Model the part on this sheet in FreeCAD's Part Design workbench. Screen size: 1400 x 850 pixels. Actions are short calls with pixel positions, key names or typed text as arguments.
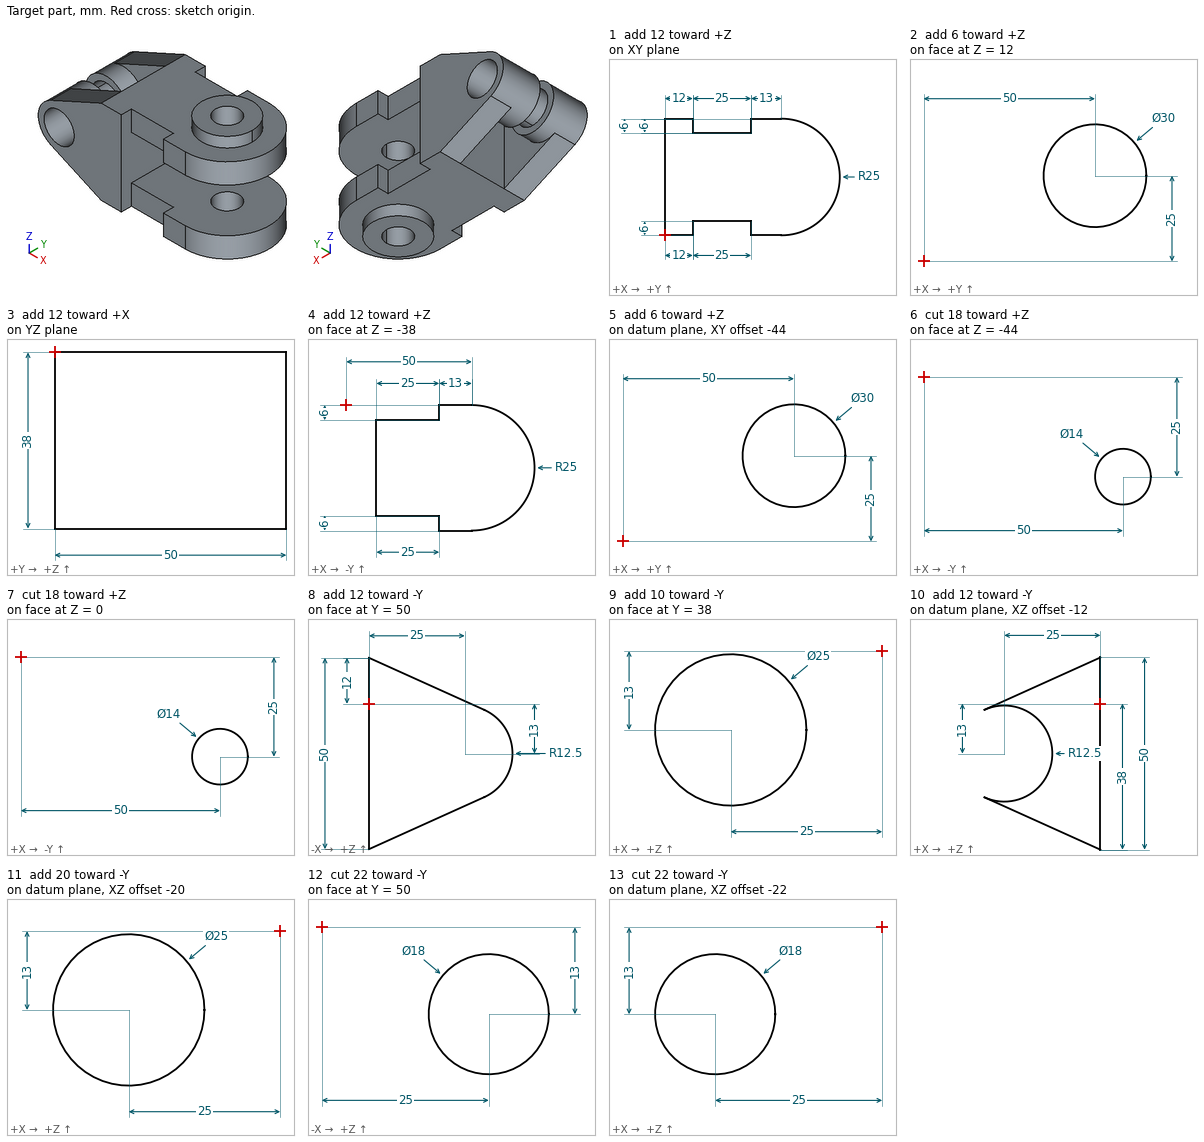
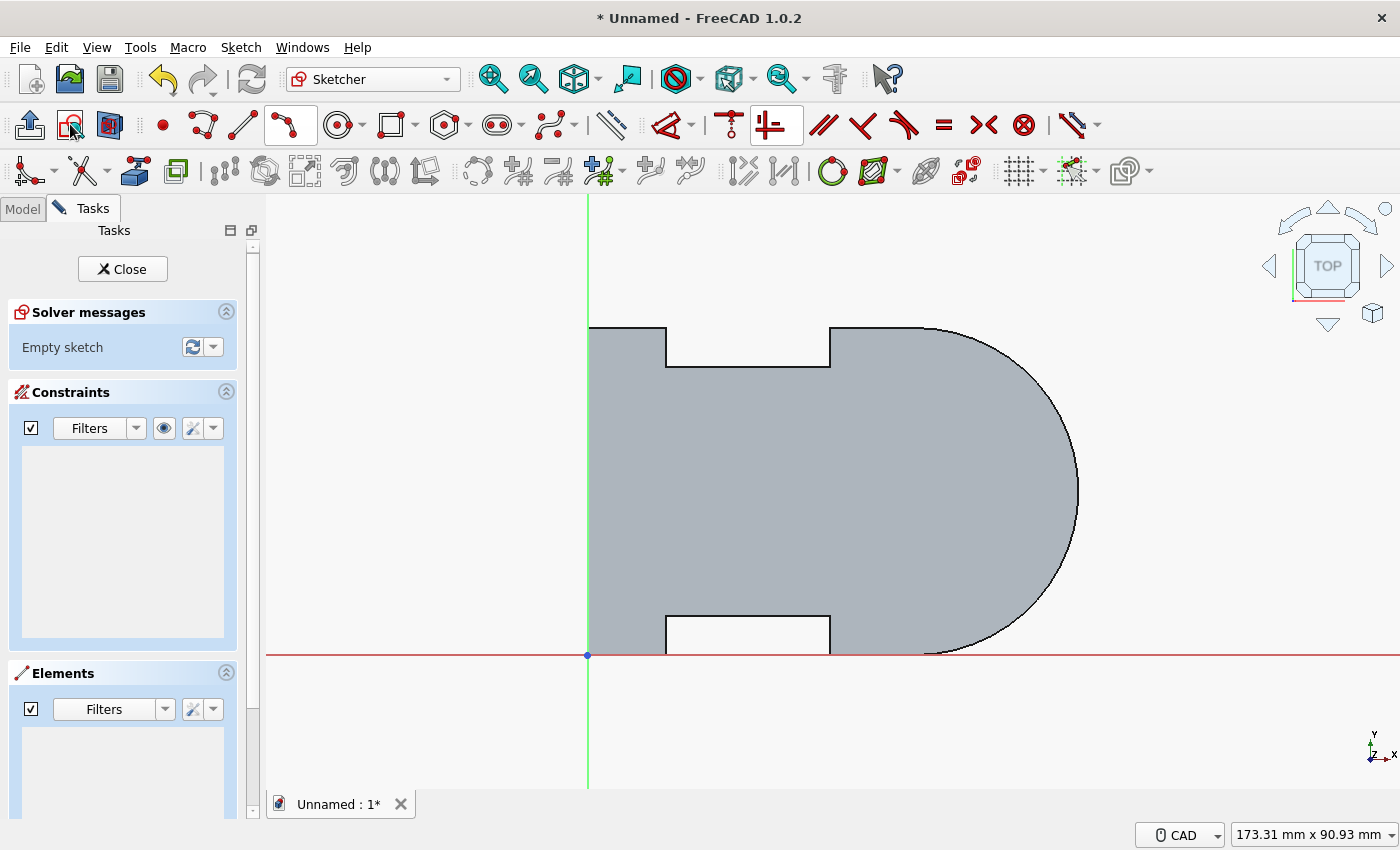
scroll(873, 591, up, 2)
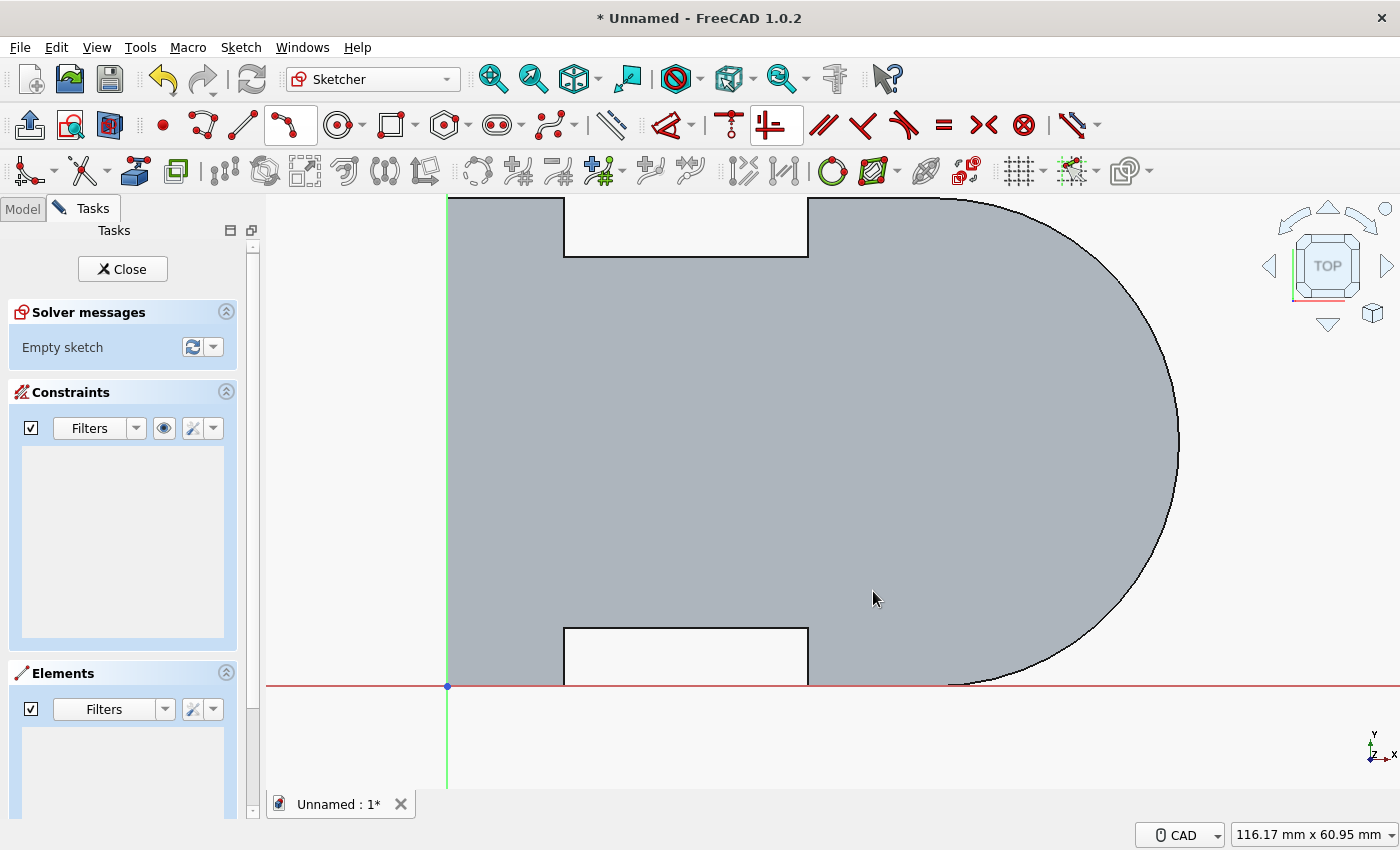
click(338, 126)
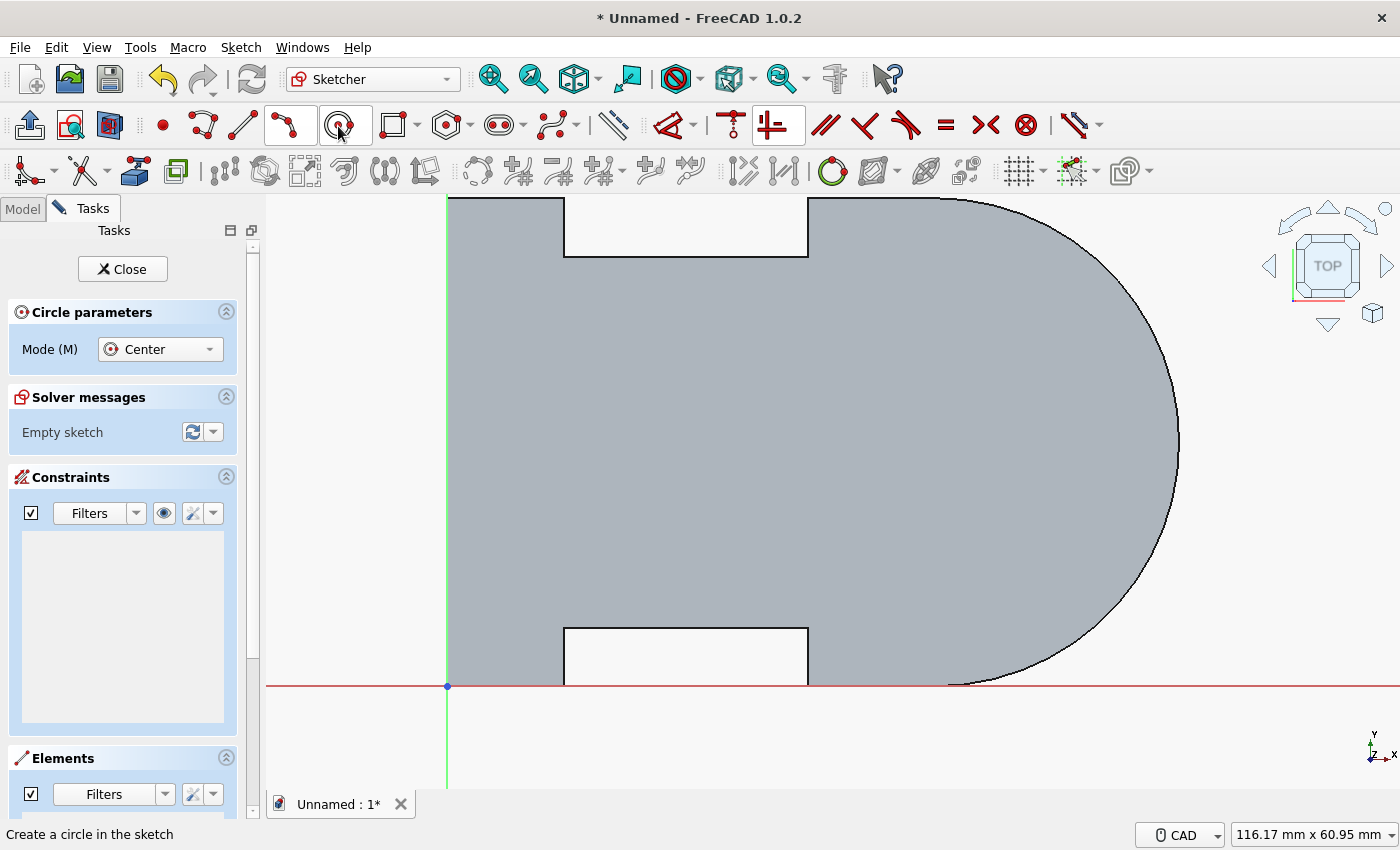
click(935, 442)
click(1039, 339)
key(Escape)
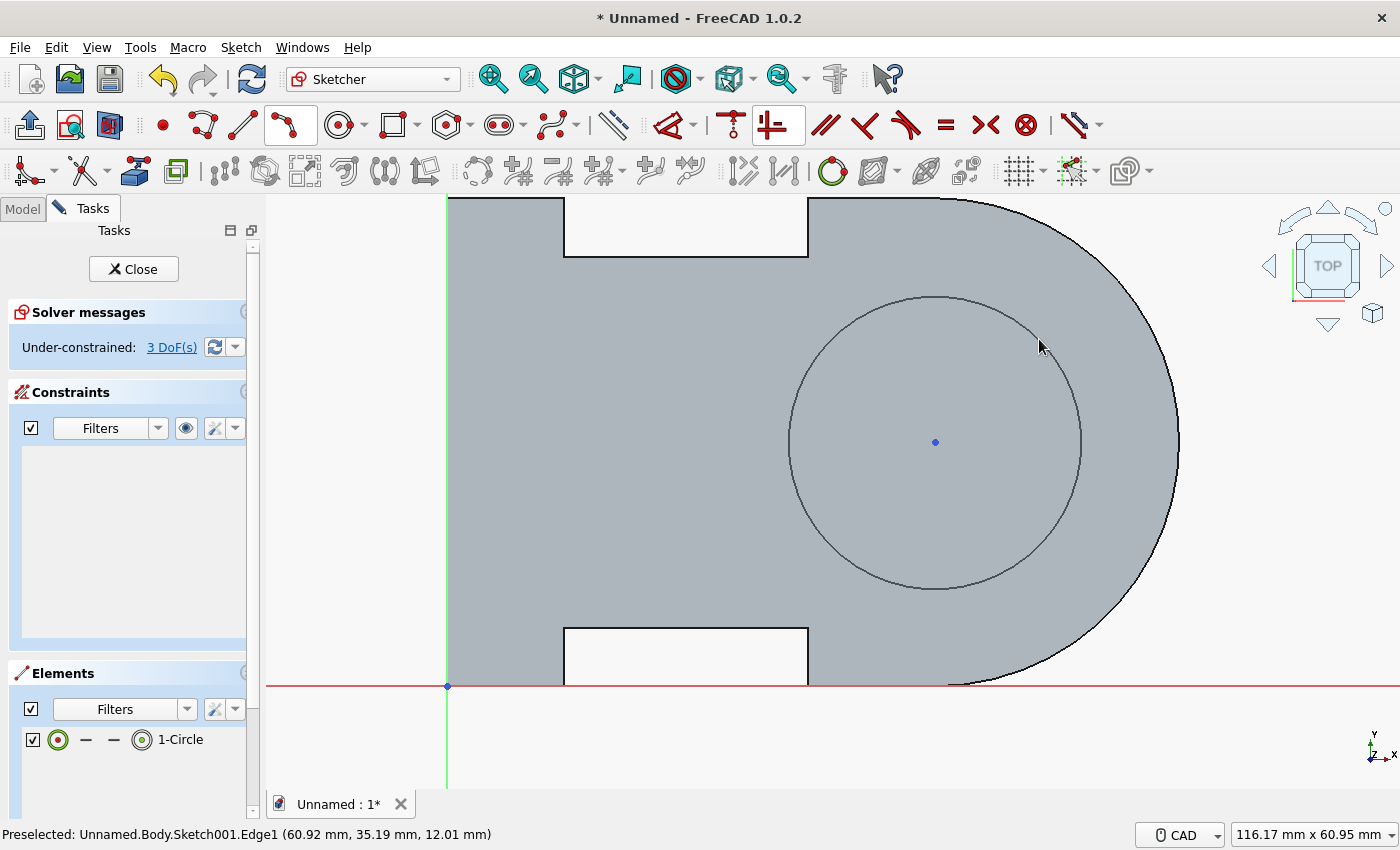
click(668, 126)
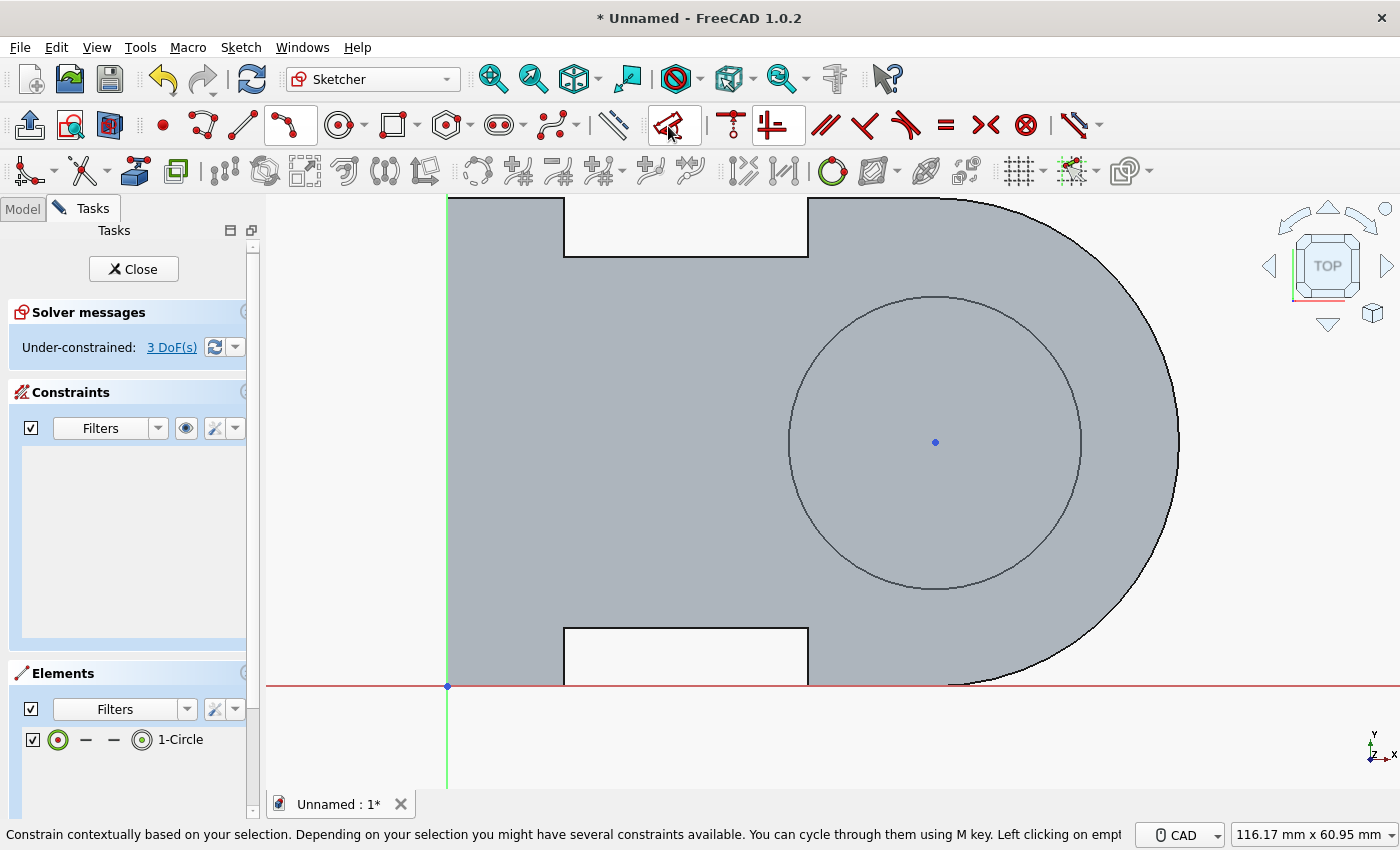
click(1038, 339)
click(1061, 316)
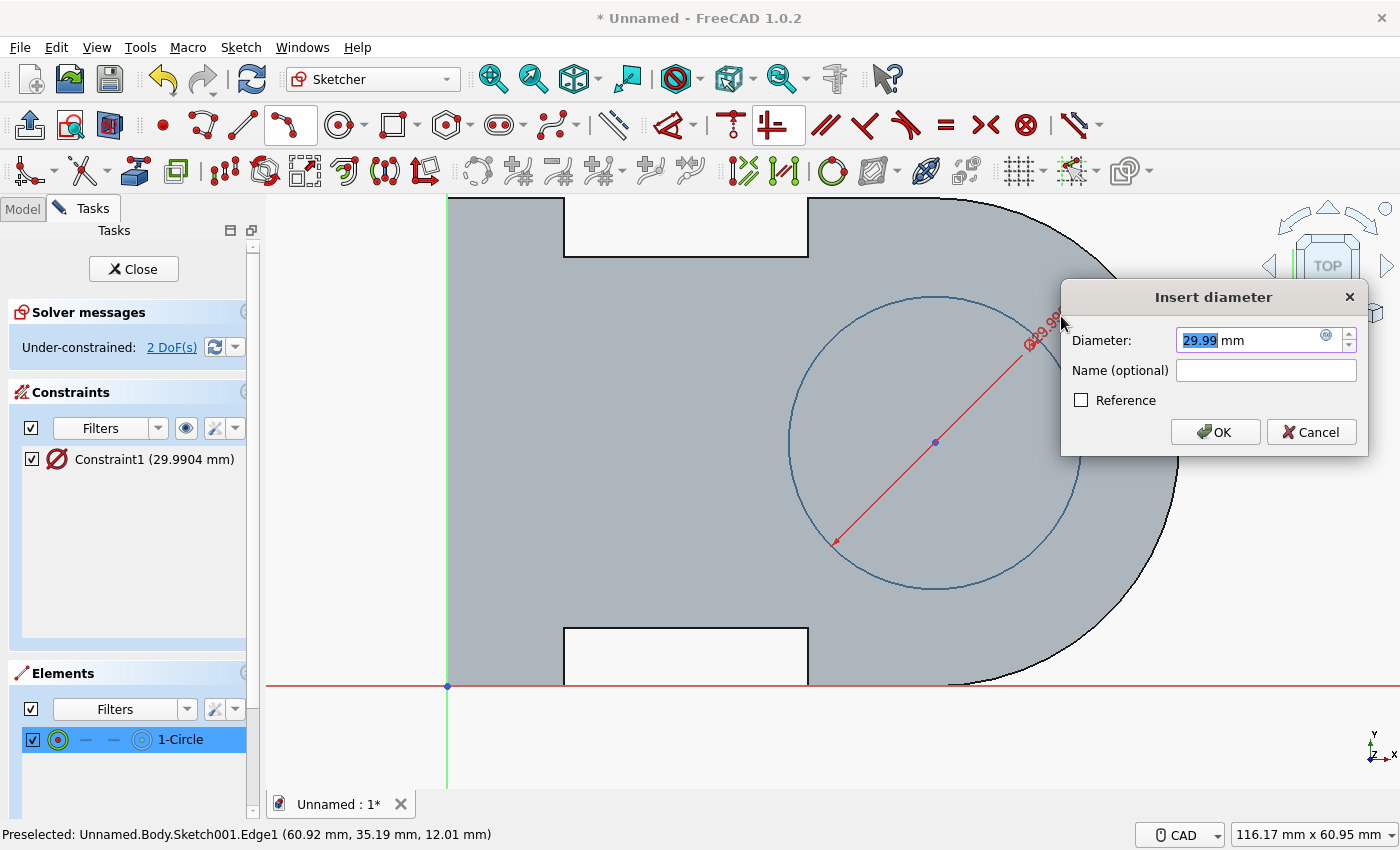
text(30)
key(Return)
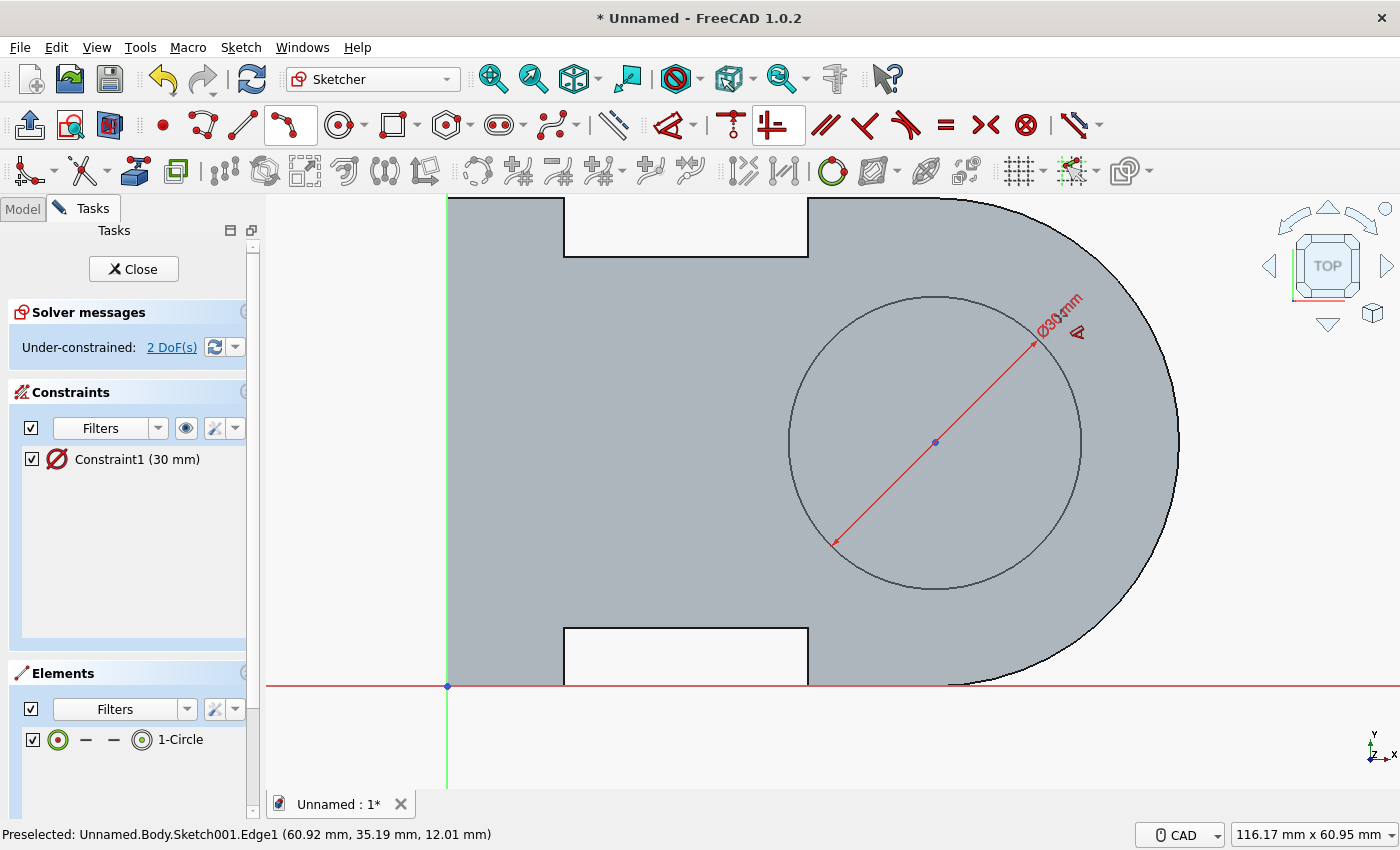
click(935, 443)
click(691, 720)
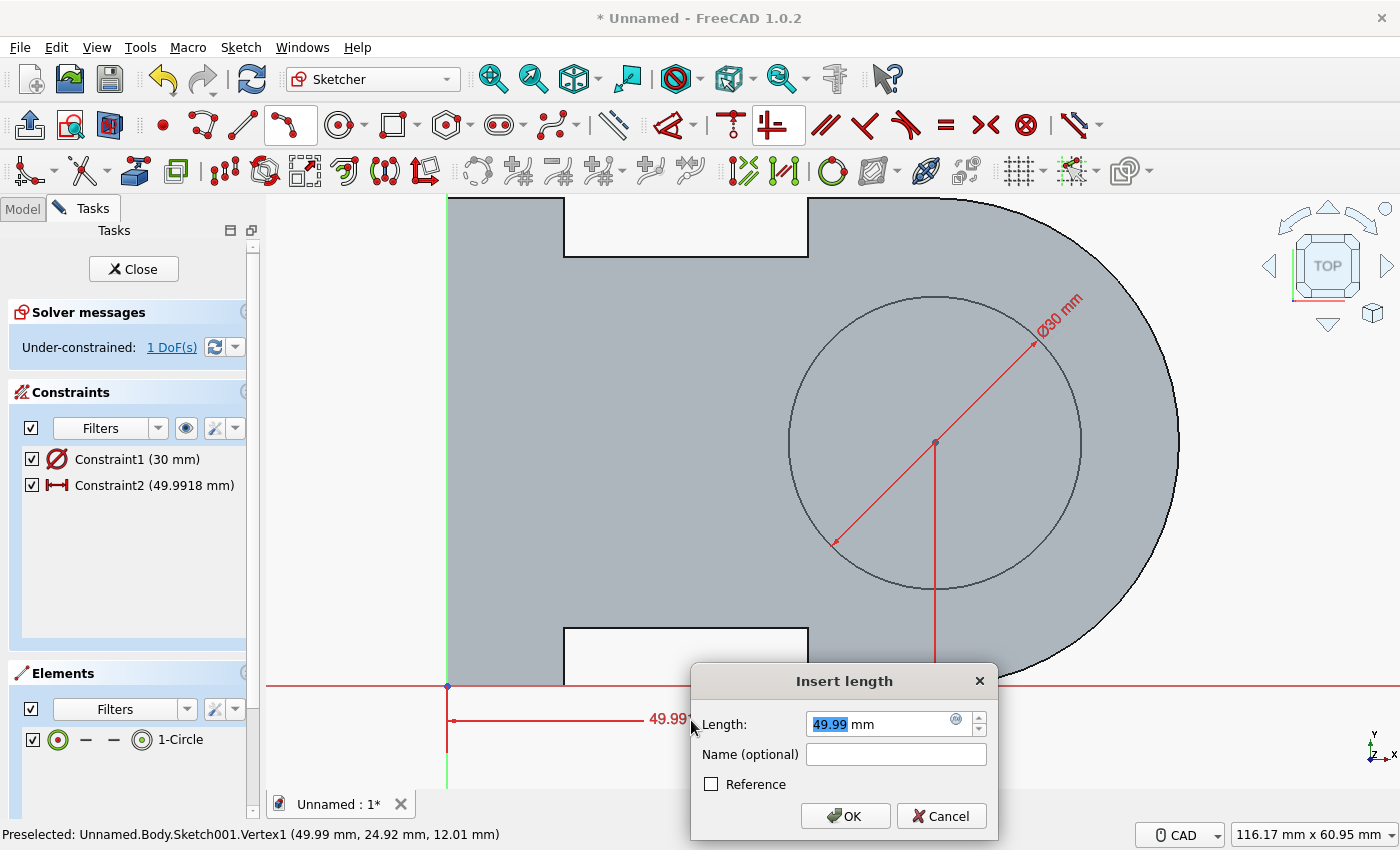
text(50)
key(Return)